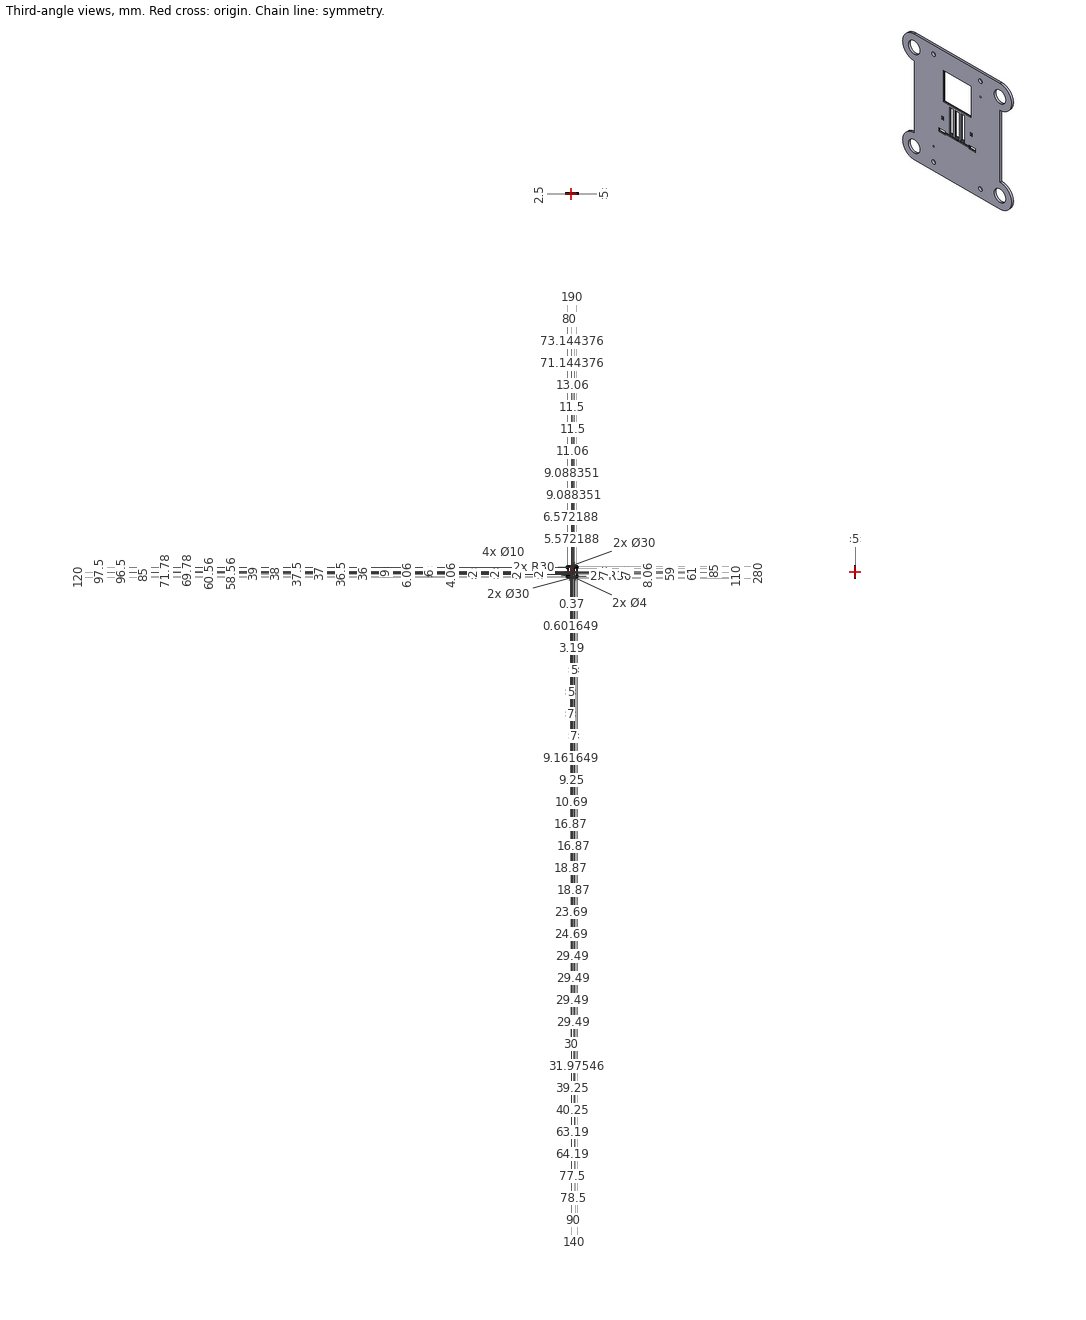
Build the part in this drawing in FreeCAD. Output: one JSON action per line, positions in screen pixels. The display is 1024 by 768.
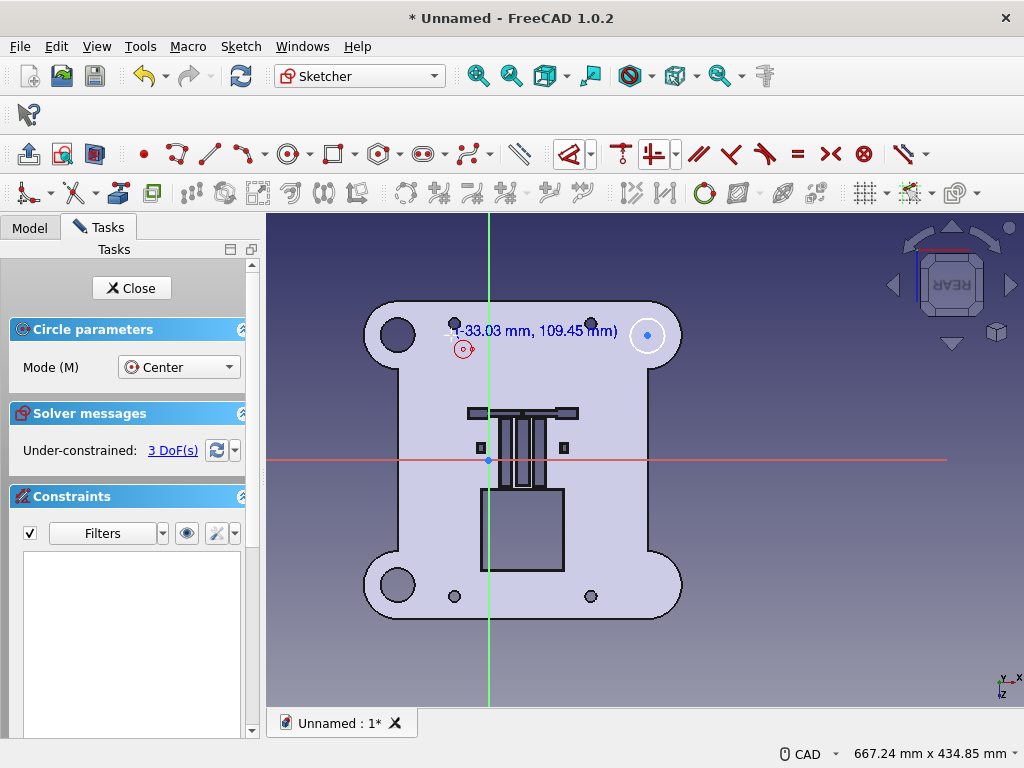
{"action": "scroll", "coordinate": [648, 585], "scroll_direction": "up", "scroll_amount": 2}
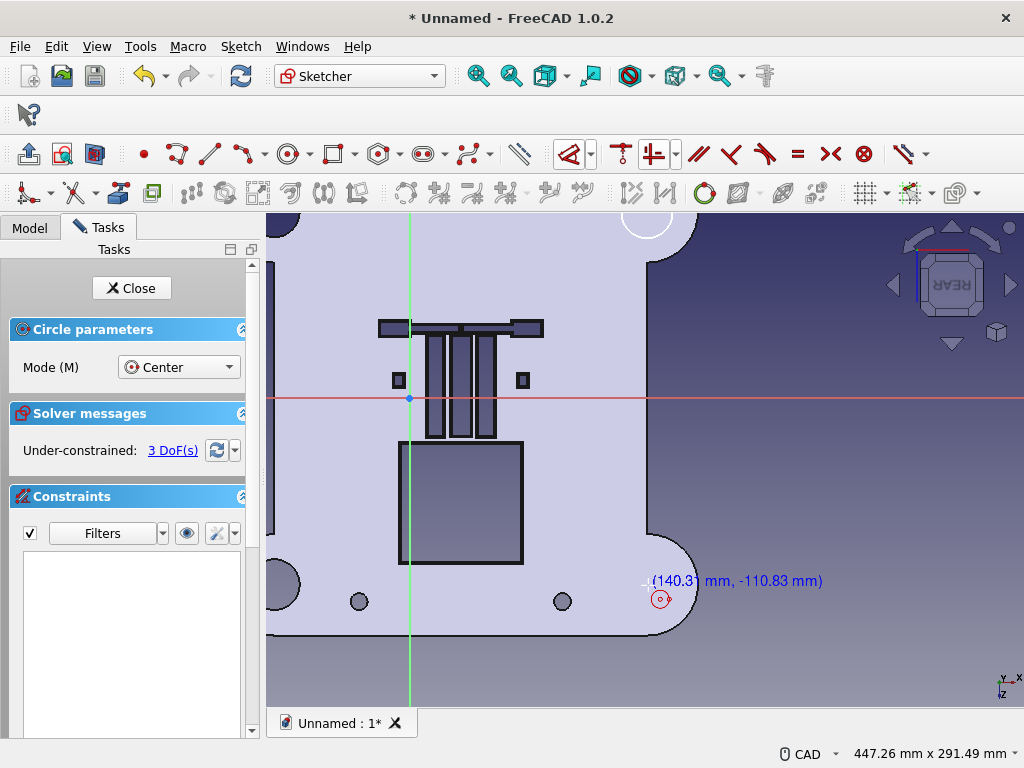
{"action": "left_click", "coordinate": [647, 585]}
{"action": "left_click", "coordinate": [665, 567]}
{"action": "key", "text": "Escape"}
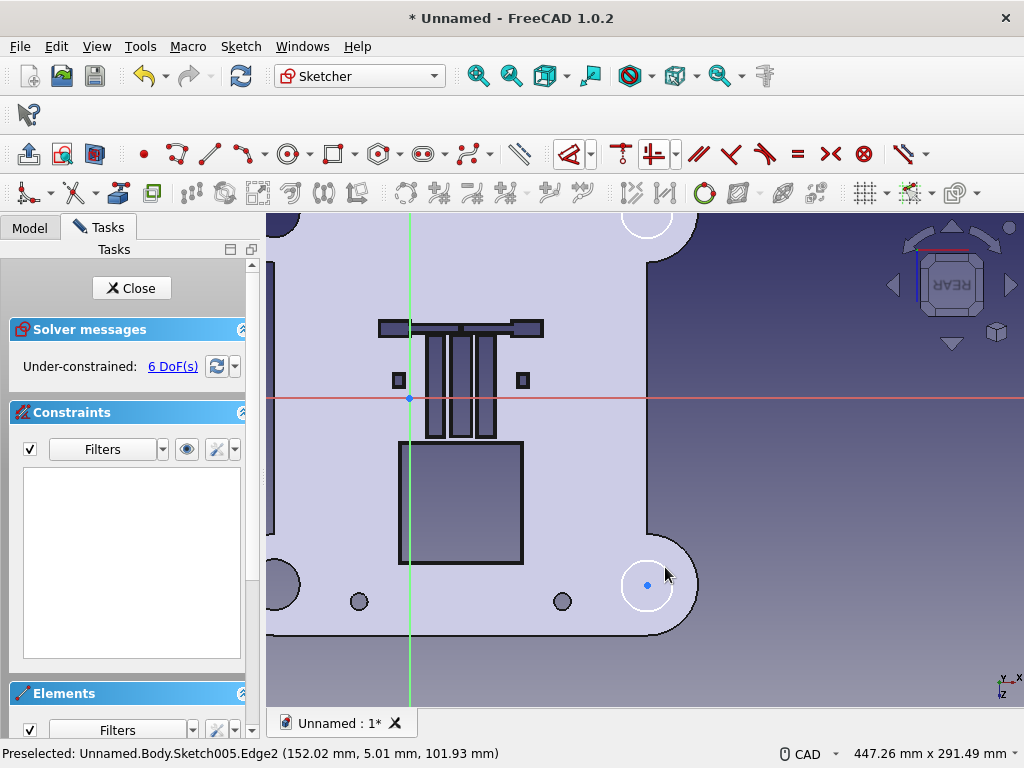
{"action": "scroll", "coordinate": [648, 585], "scroll_direction": "down", "scroll_amount": 2}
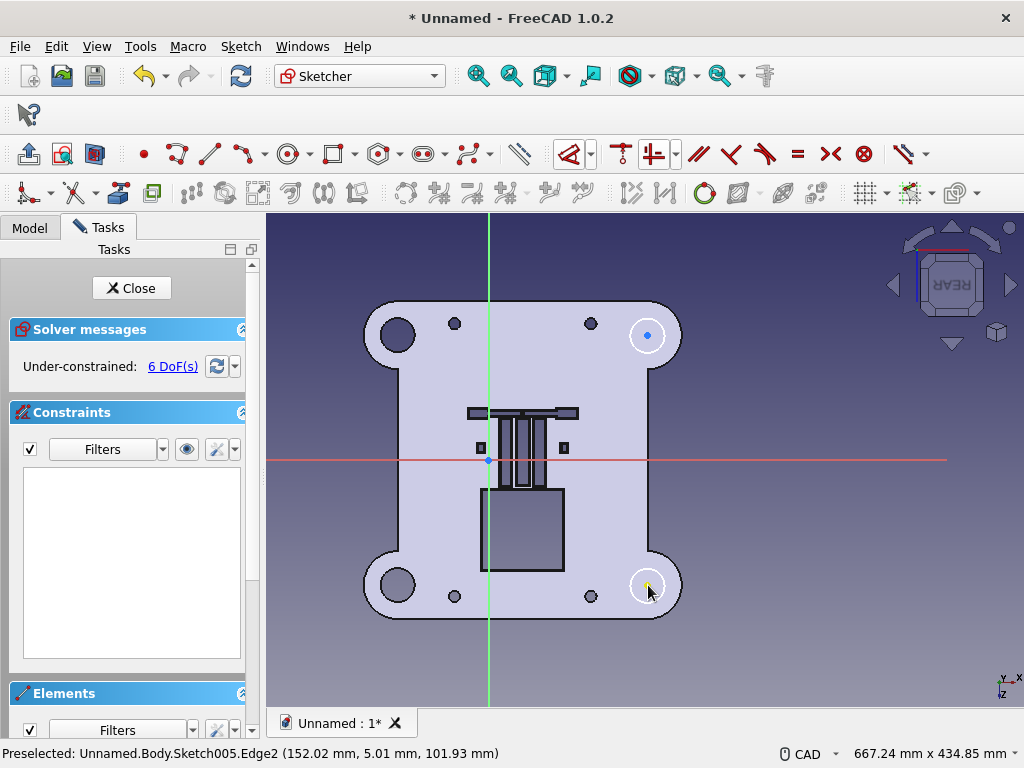
{"action": "left_click", "coordinate": [660, 324]}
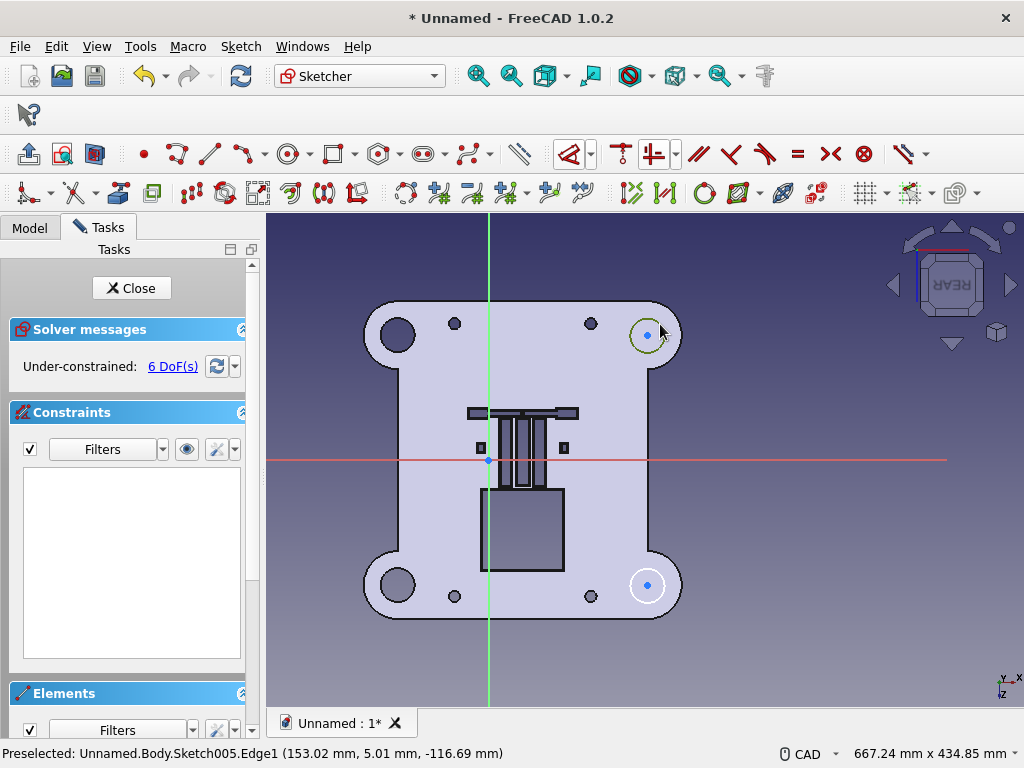
{"action": "left_click", "coordinate": [660, 574]}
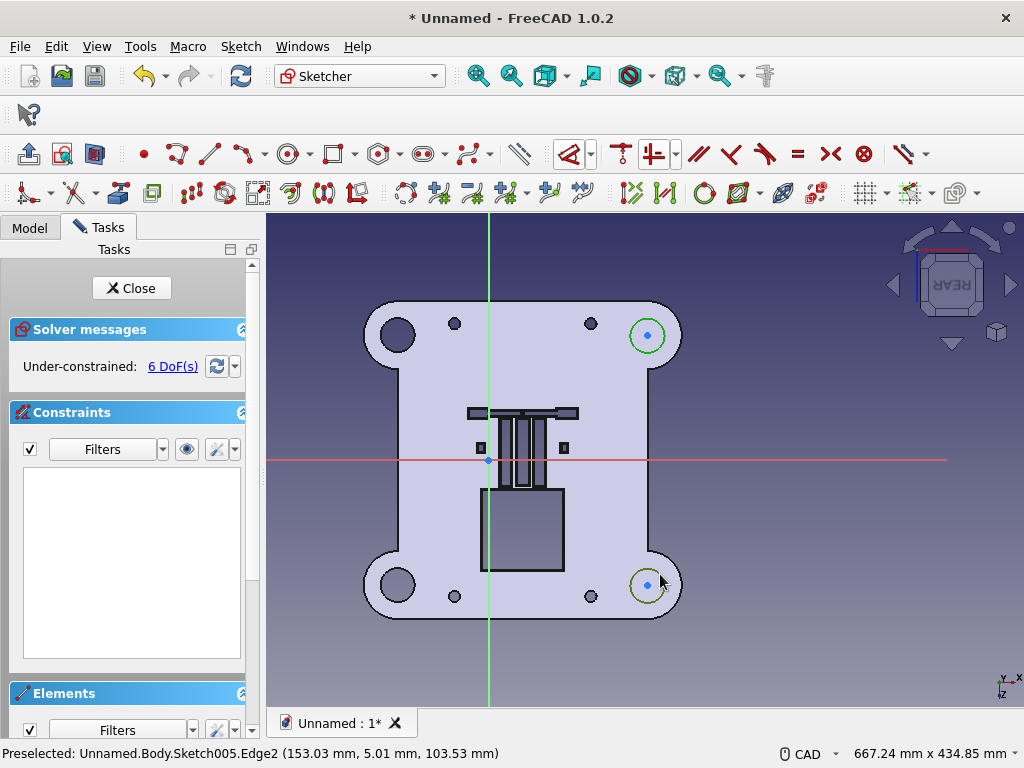
{"action": "left_click", "coordinate": [798, 154]}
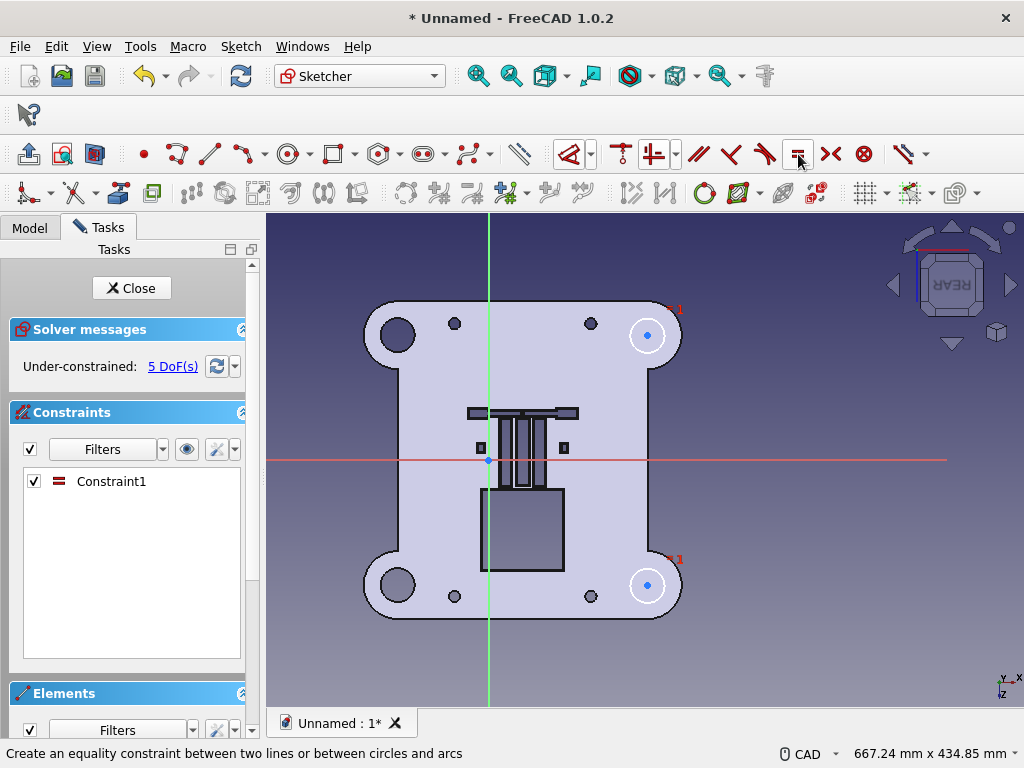
{"action": "left_click", "coordinate": [647, 336]}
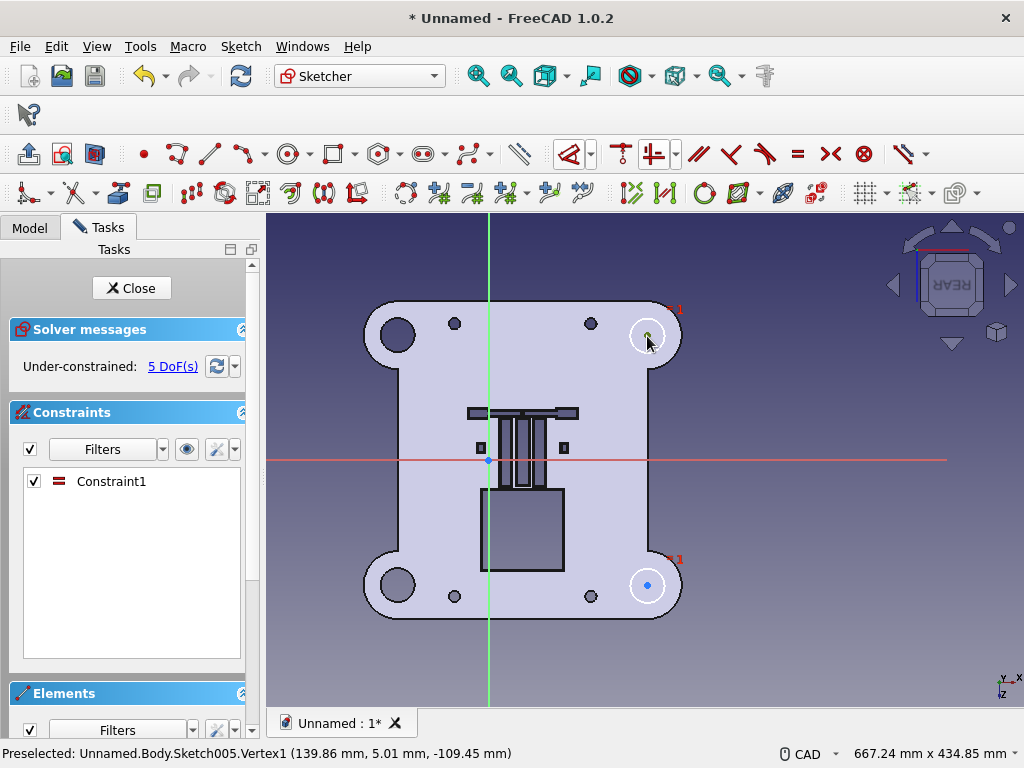
{"action": "left_click", "coordinate": [647, 586]}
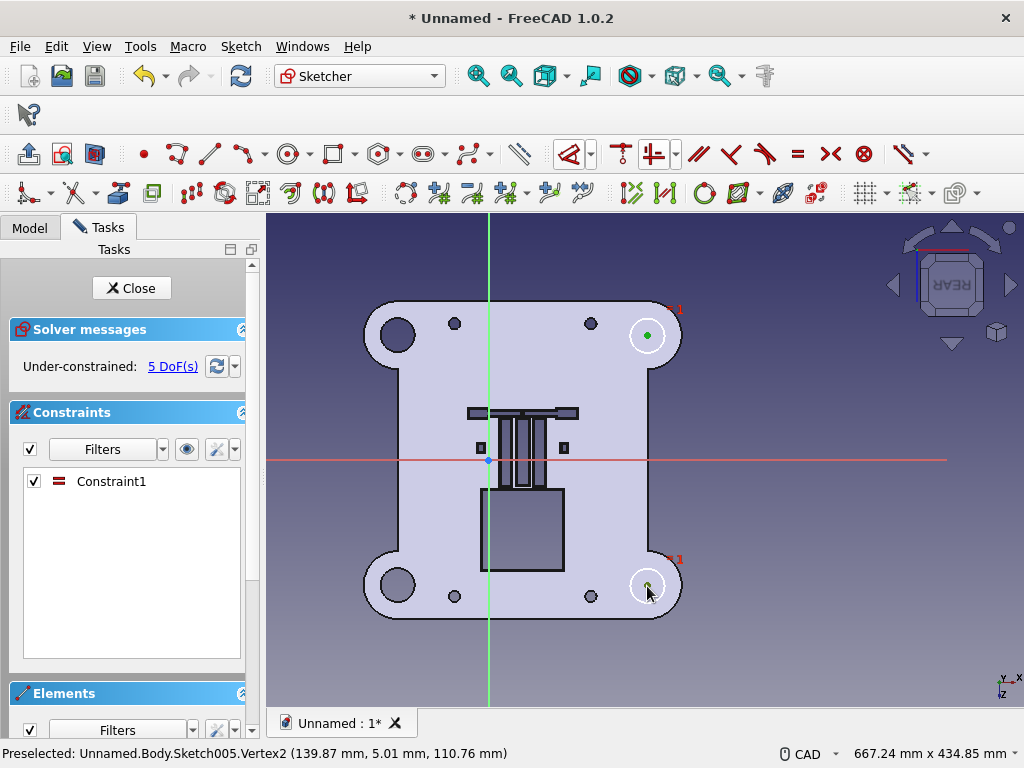
{"action": "left_click", "coordinate": [334, 460]}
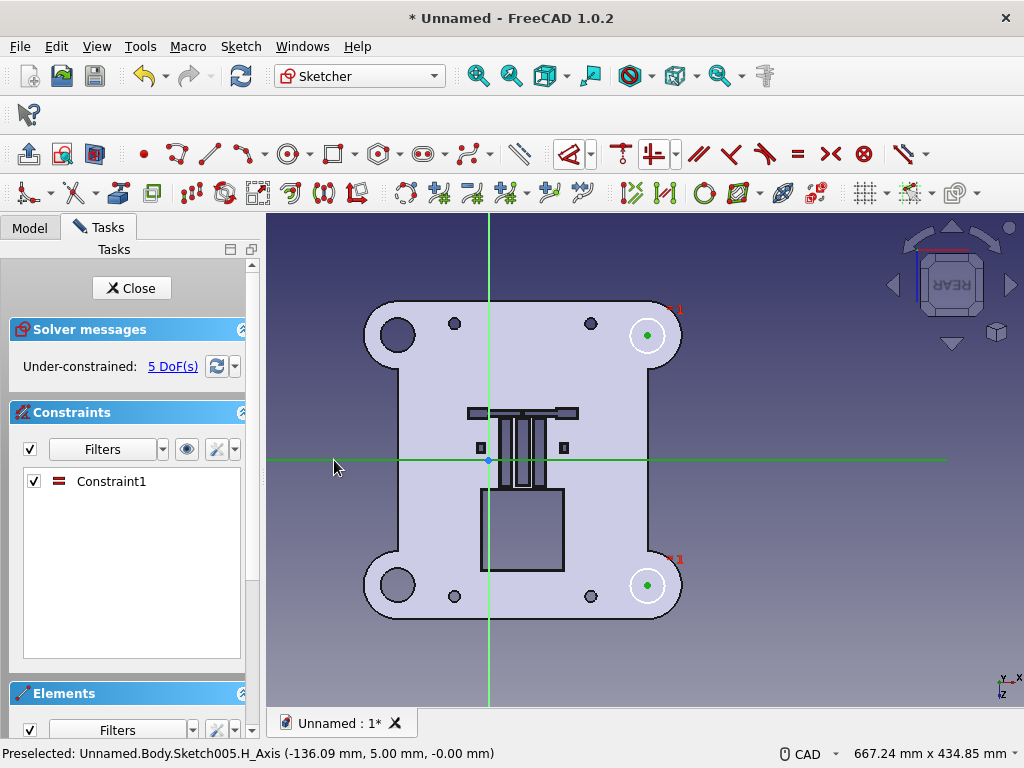
{"action": "left_click", "coordinate": [831, 154]}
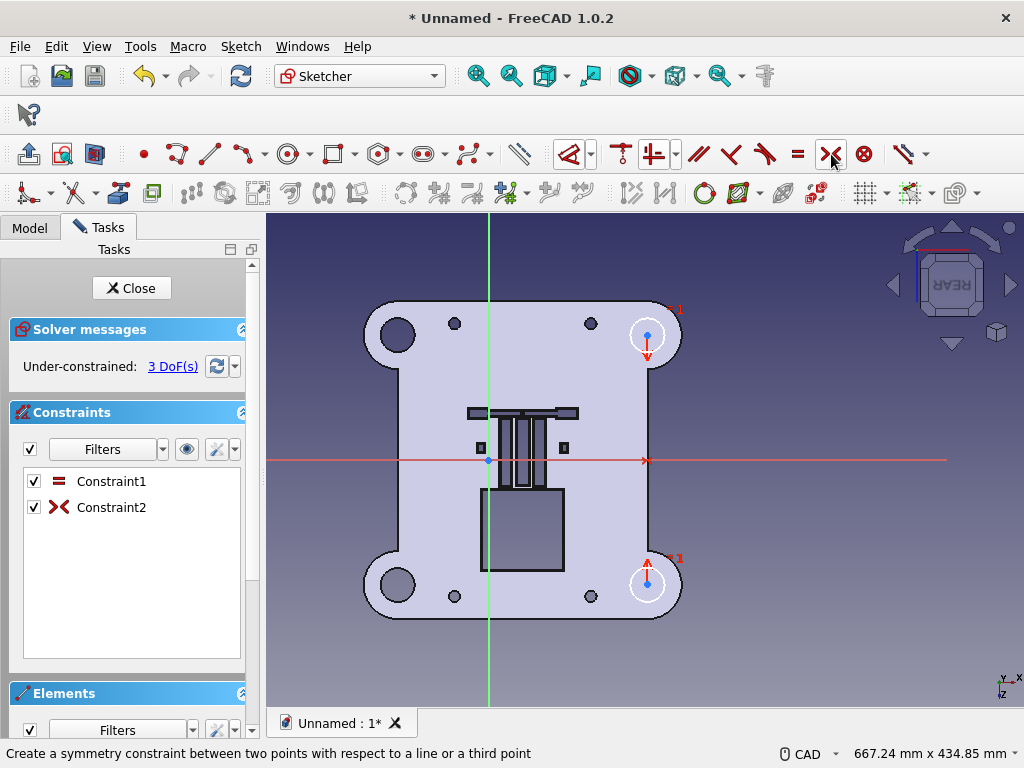
{"action": "left_click", "coordinate": [660, 323]}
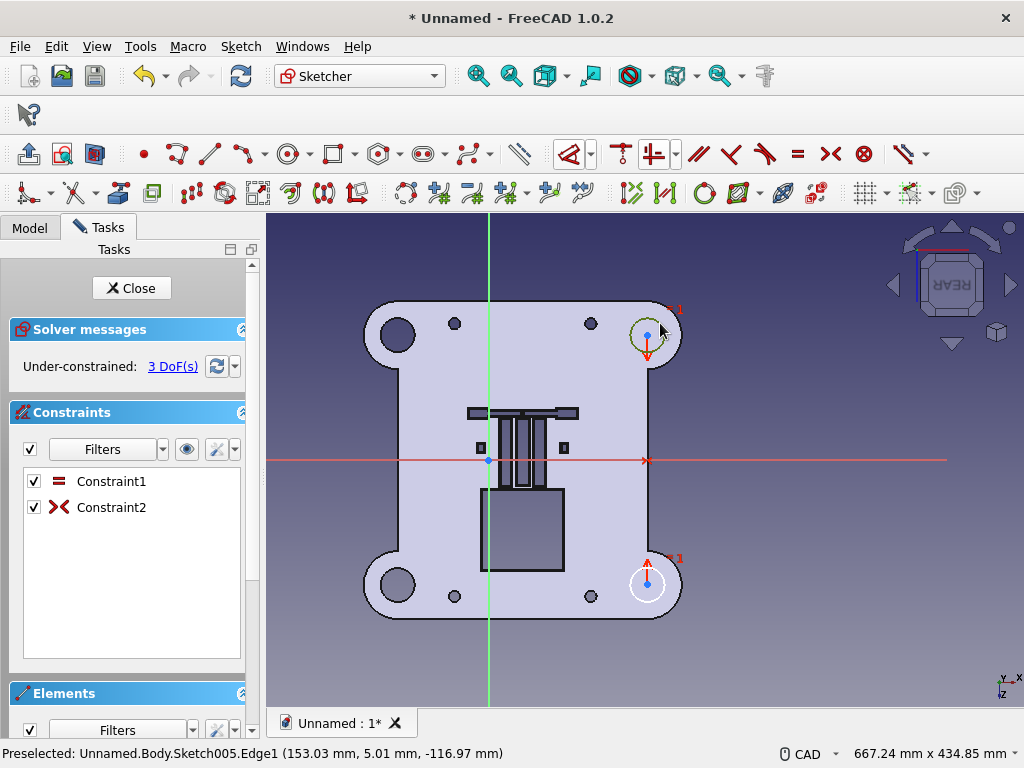
{"action": "key", "text": "k o"}